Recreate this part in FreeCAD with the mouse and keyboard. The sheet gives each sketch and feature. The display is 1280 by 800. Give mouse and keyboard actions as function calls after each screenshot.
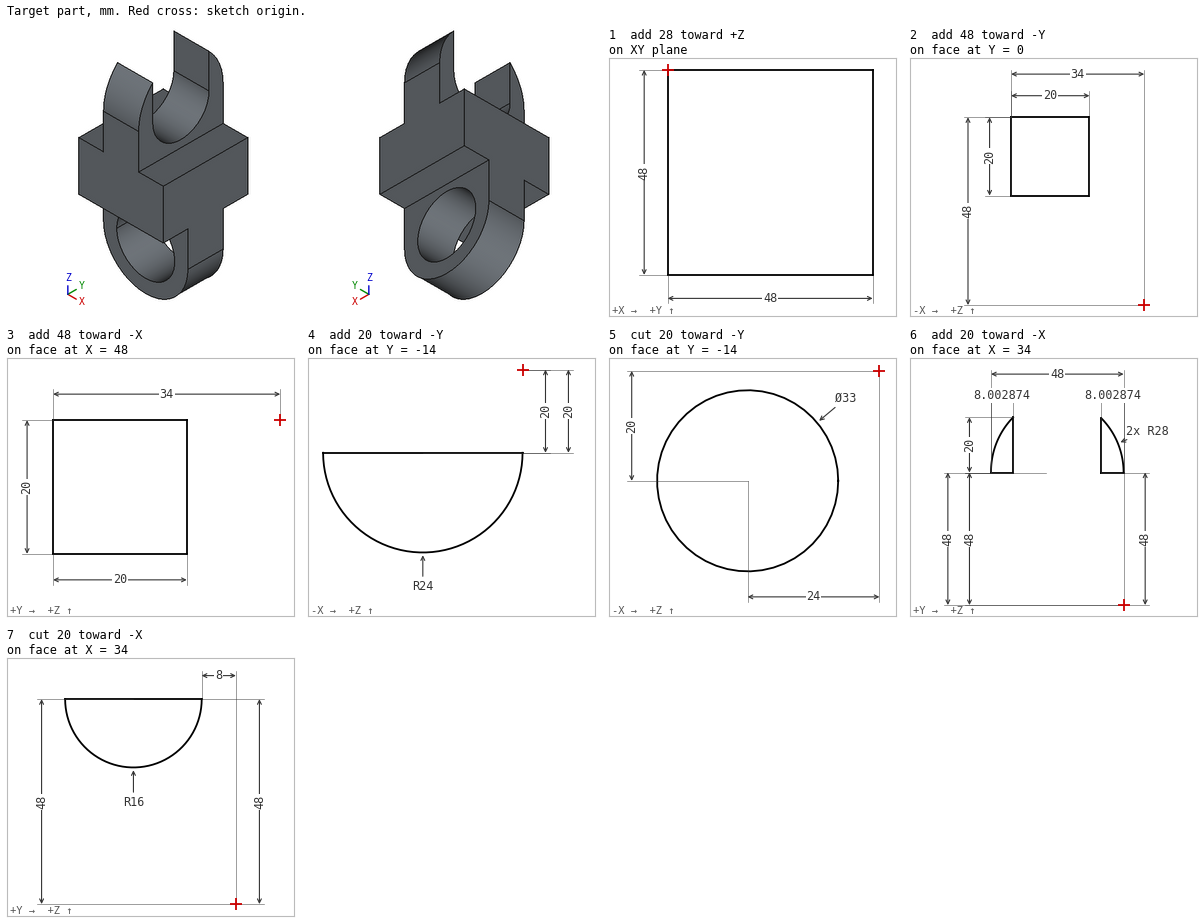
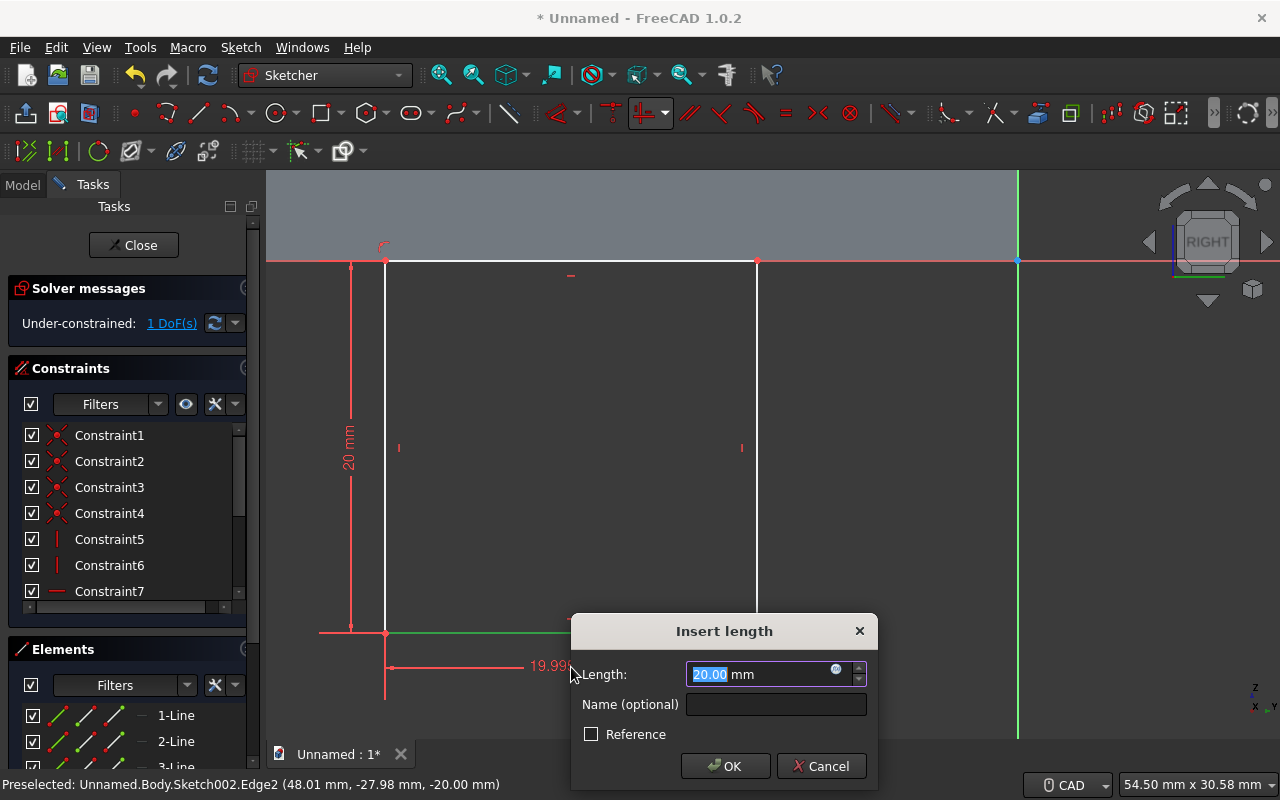
text(20)
key(Return)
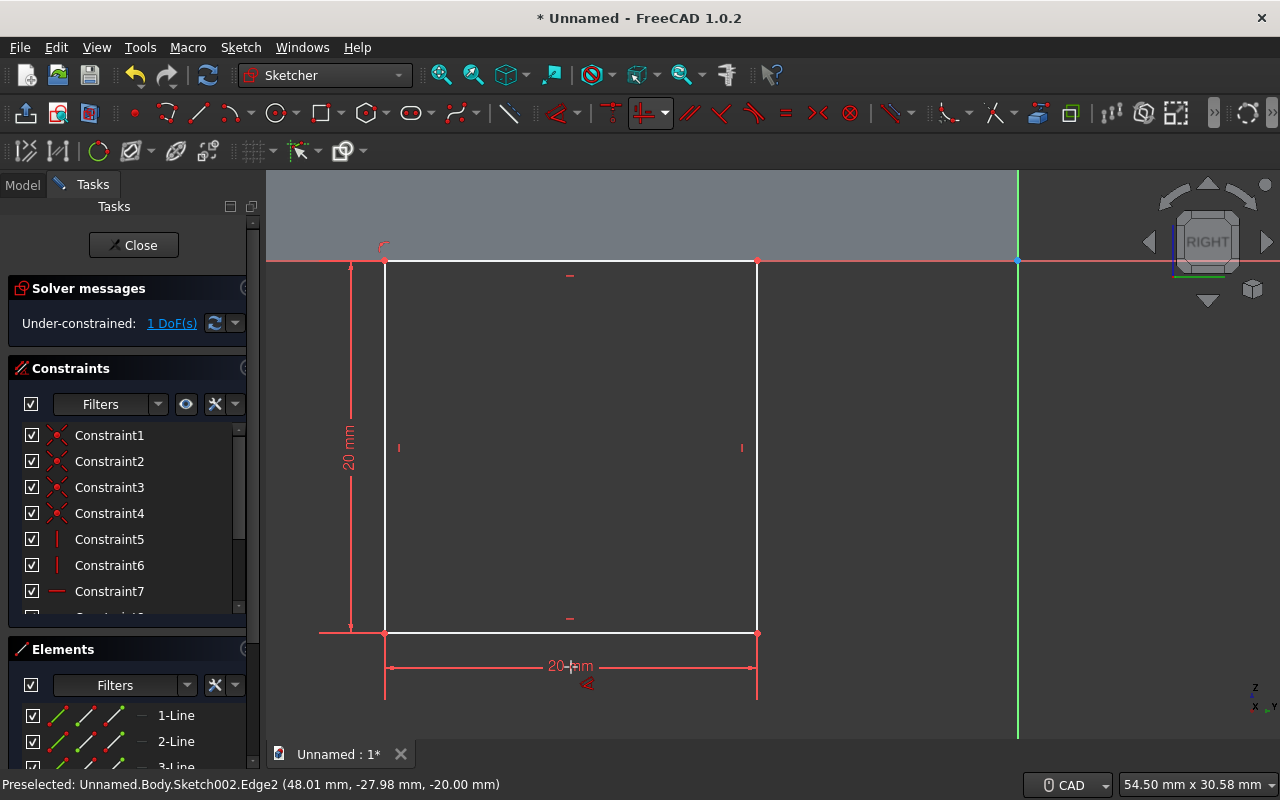
click(385, 261)
click(701, 227)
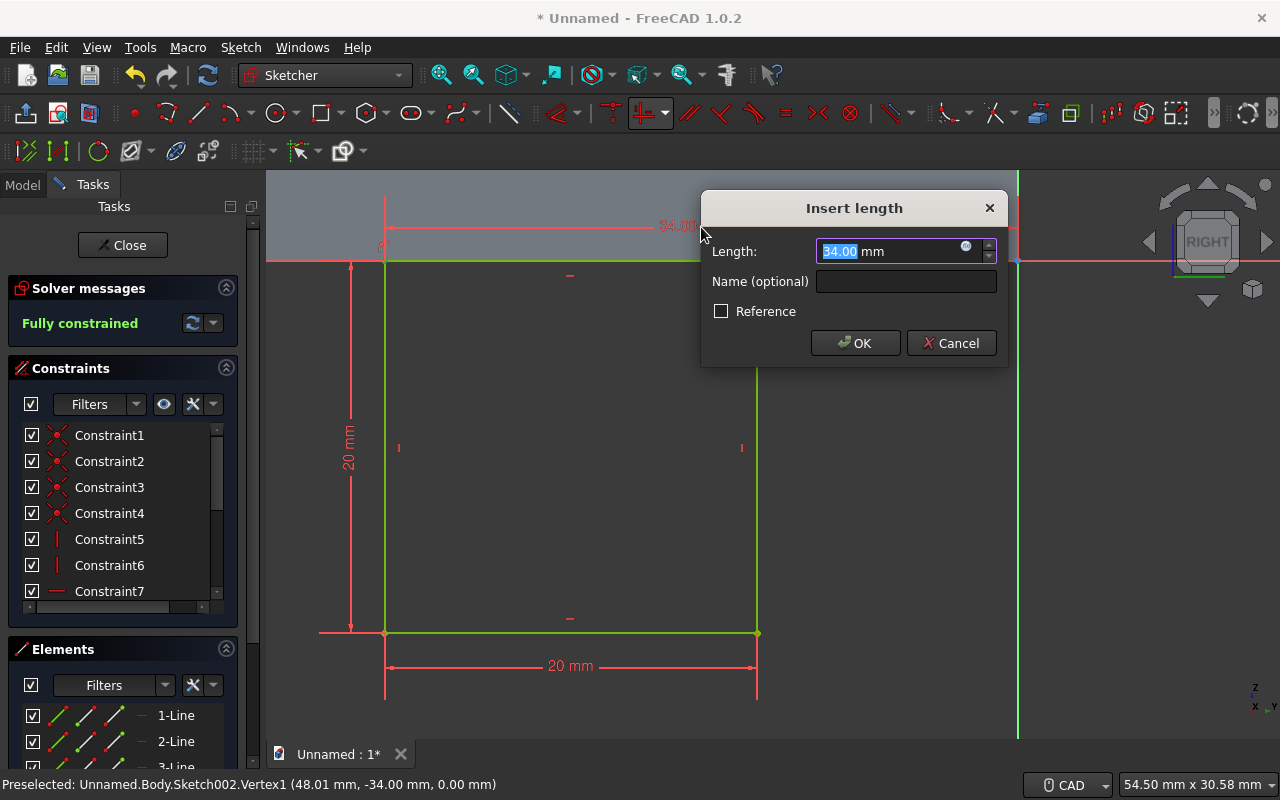
text(34)
key(Return)
key(Escape)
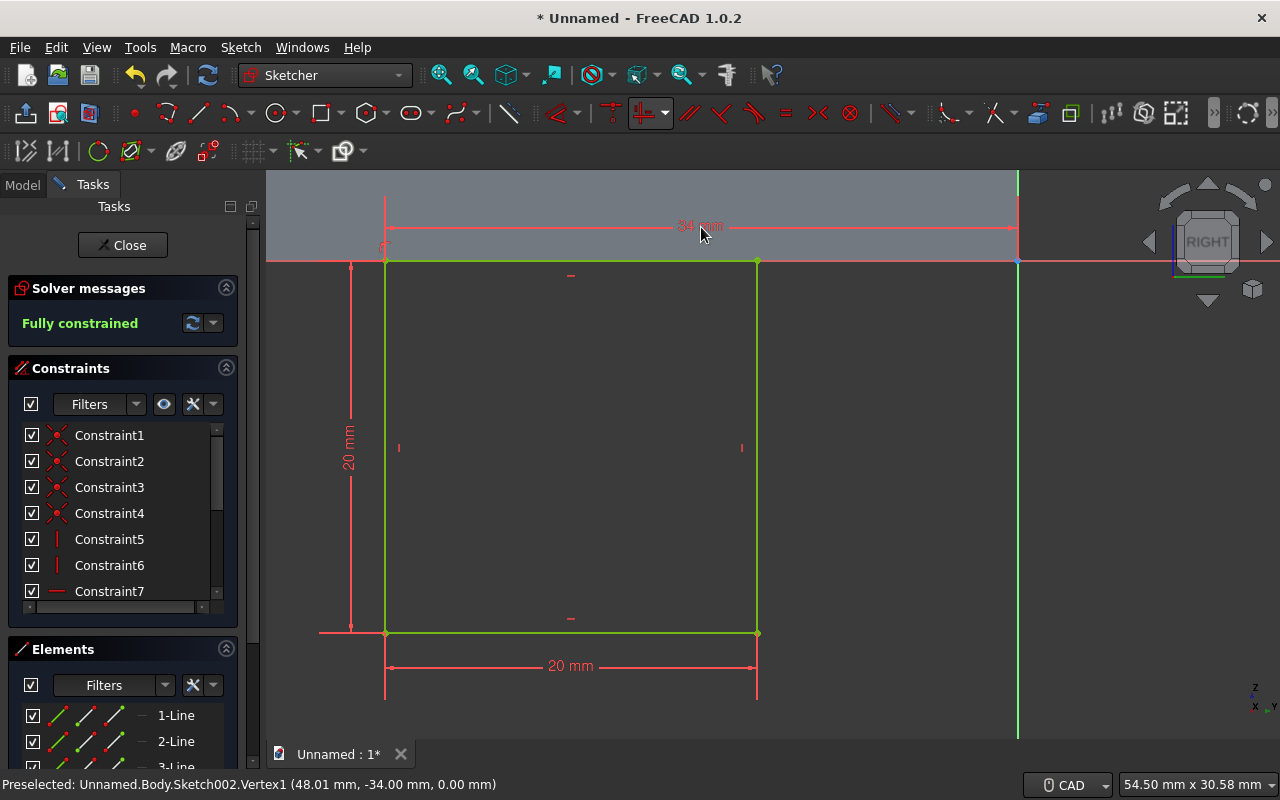
click(123, 245)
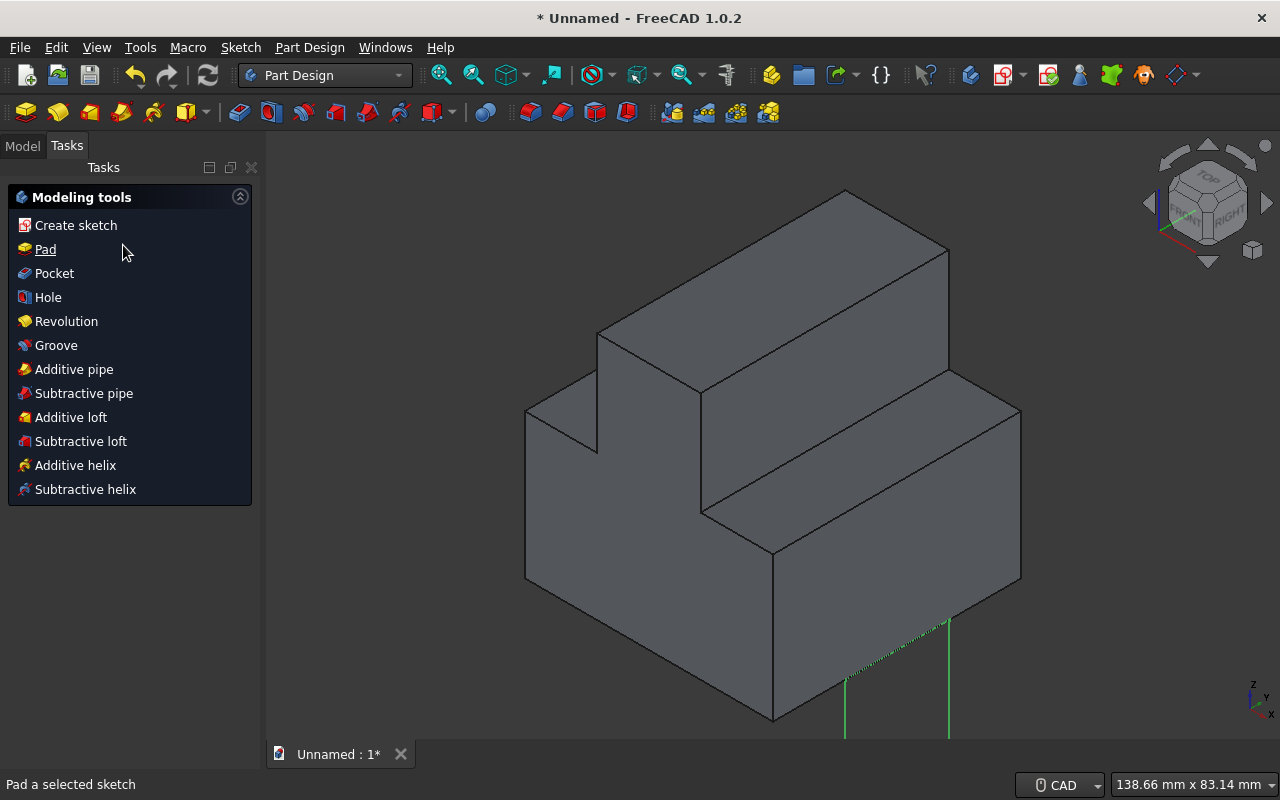
click(26, 112)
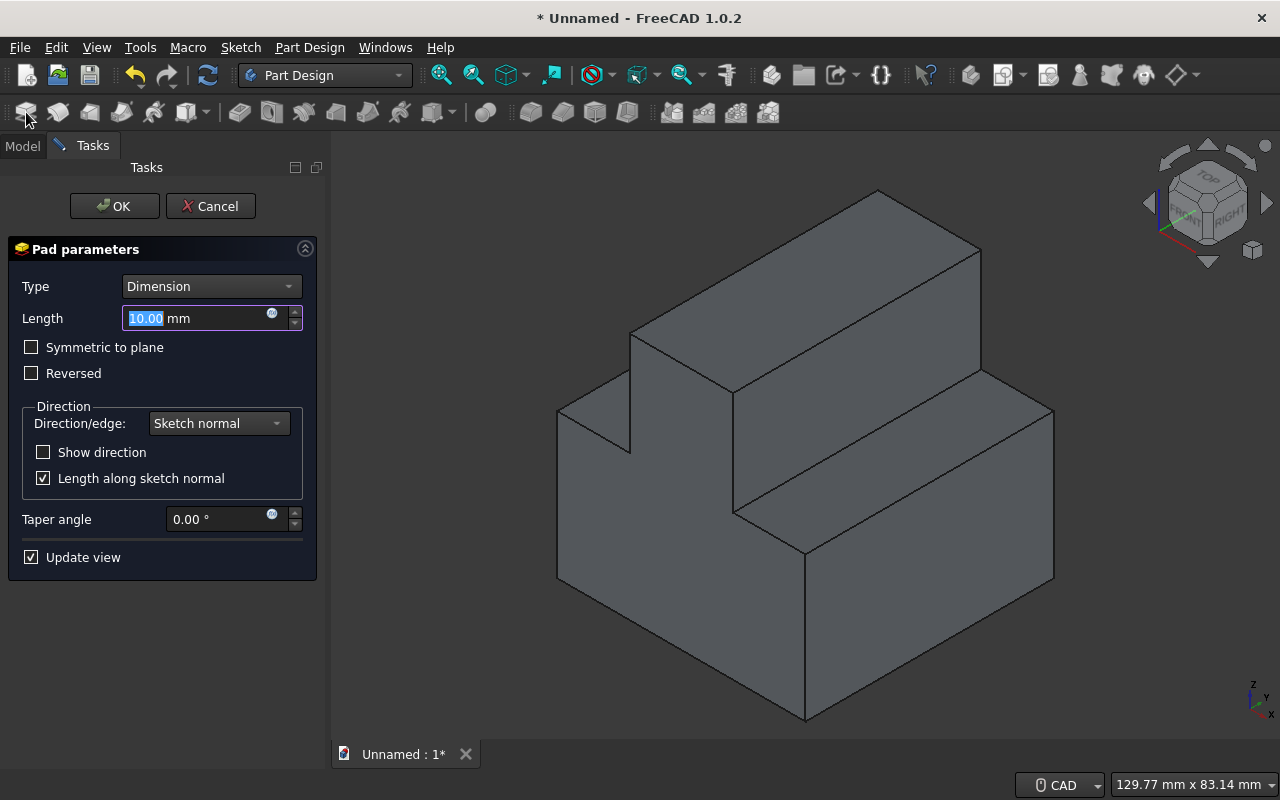
text(48)
key(Tab)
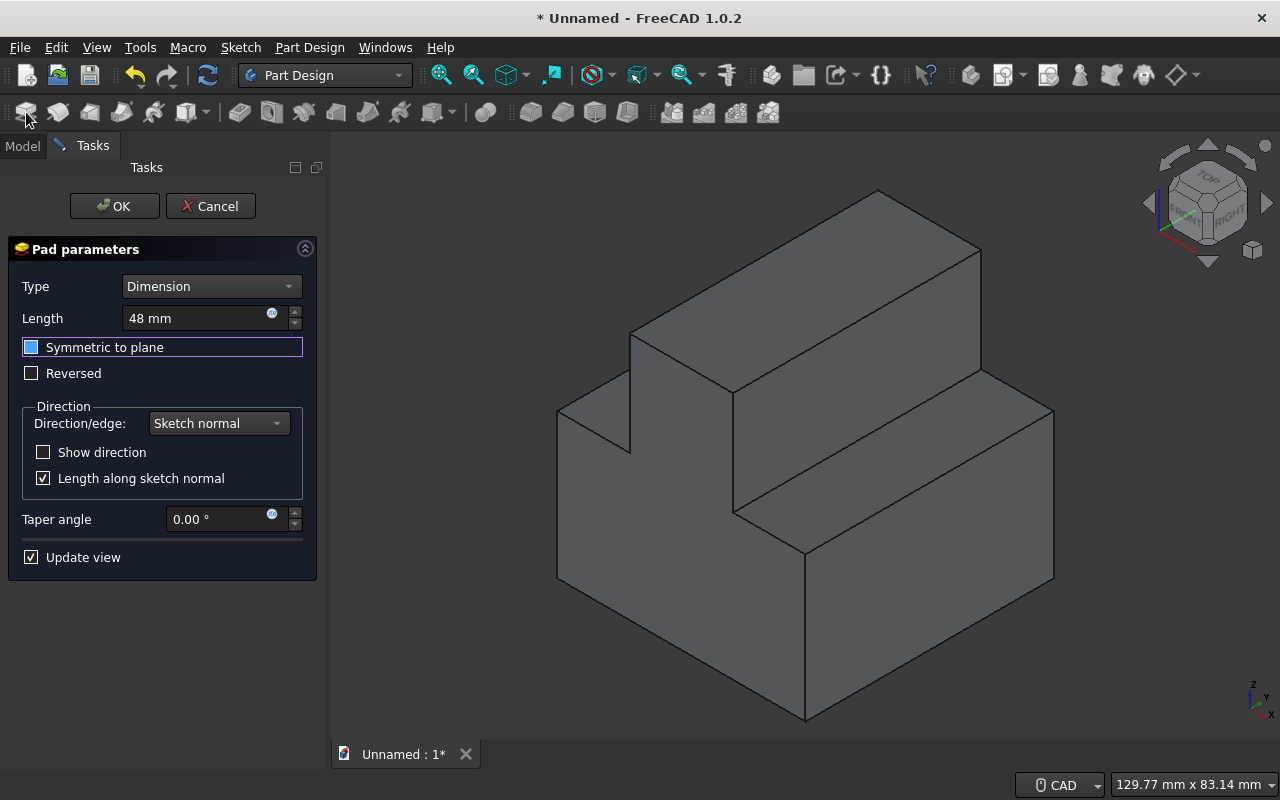
click(30, 373)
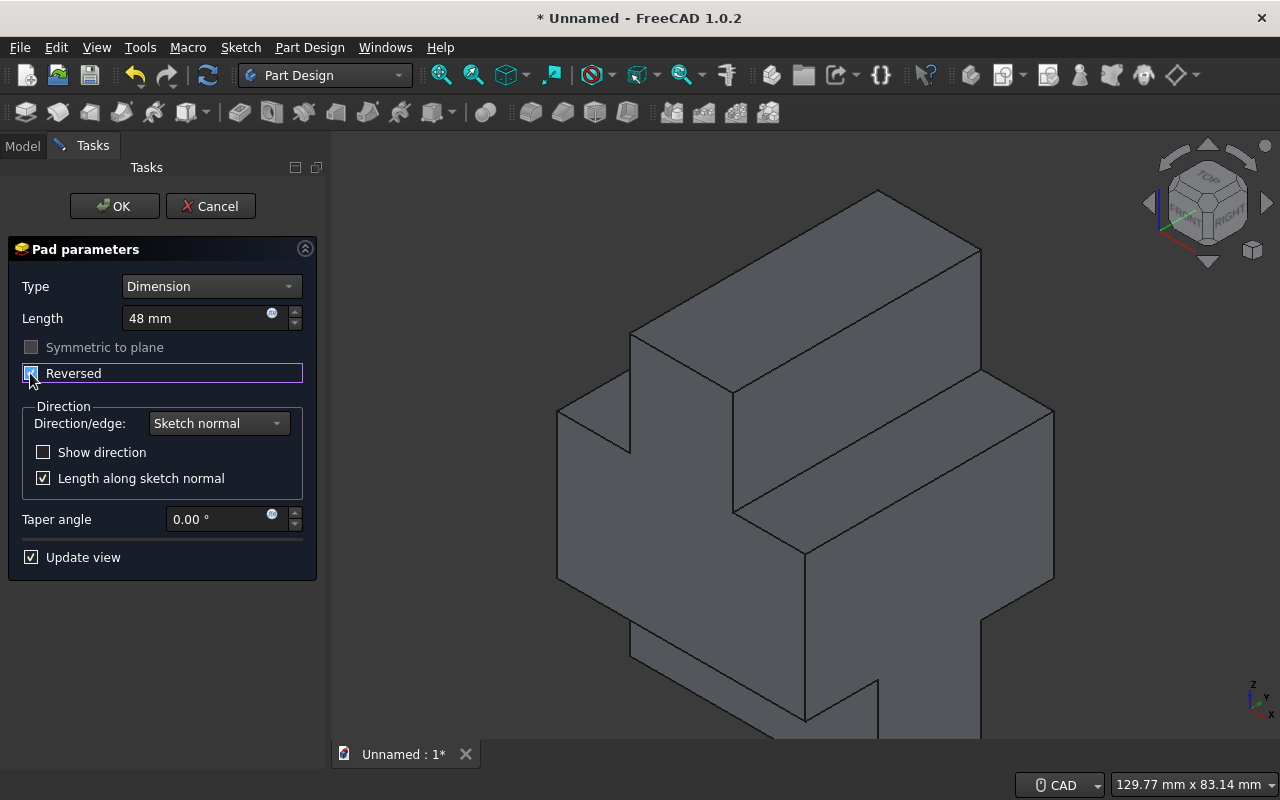
click(115, 206)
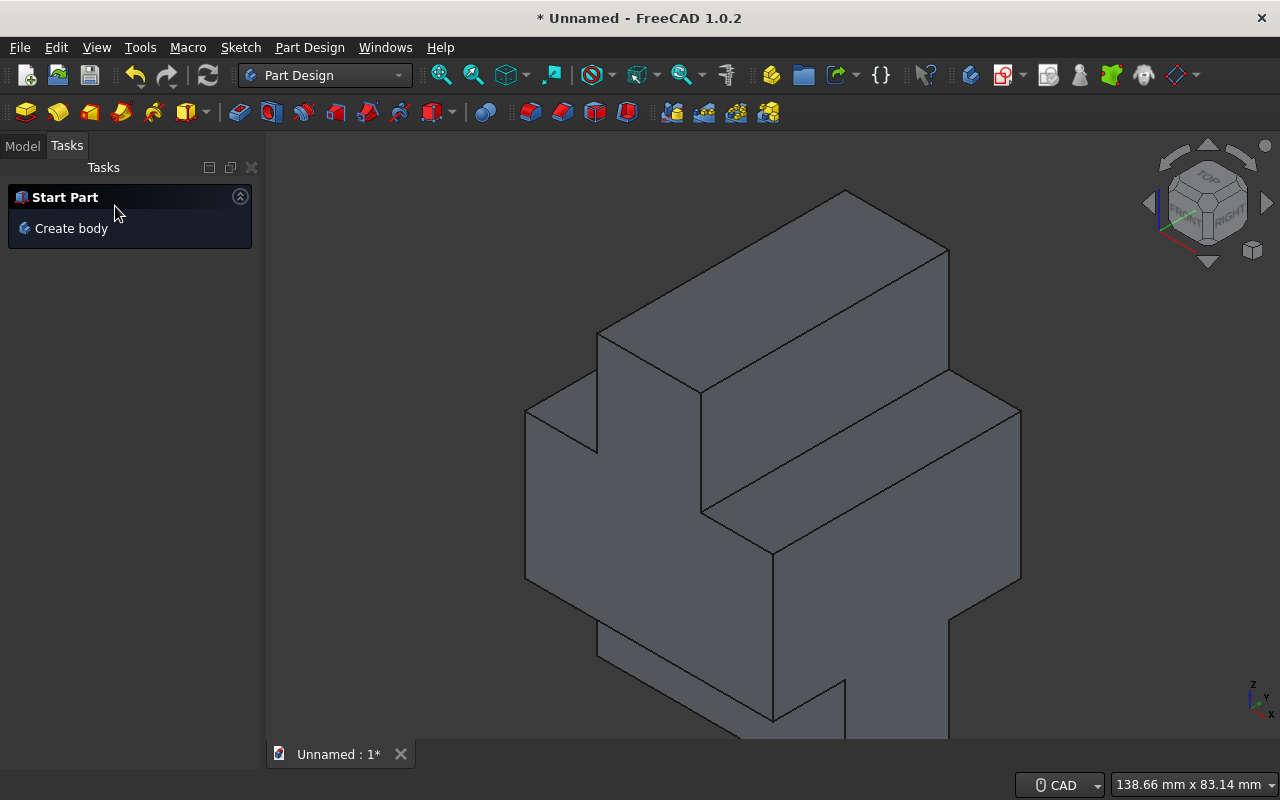
click(442, 76)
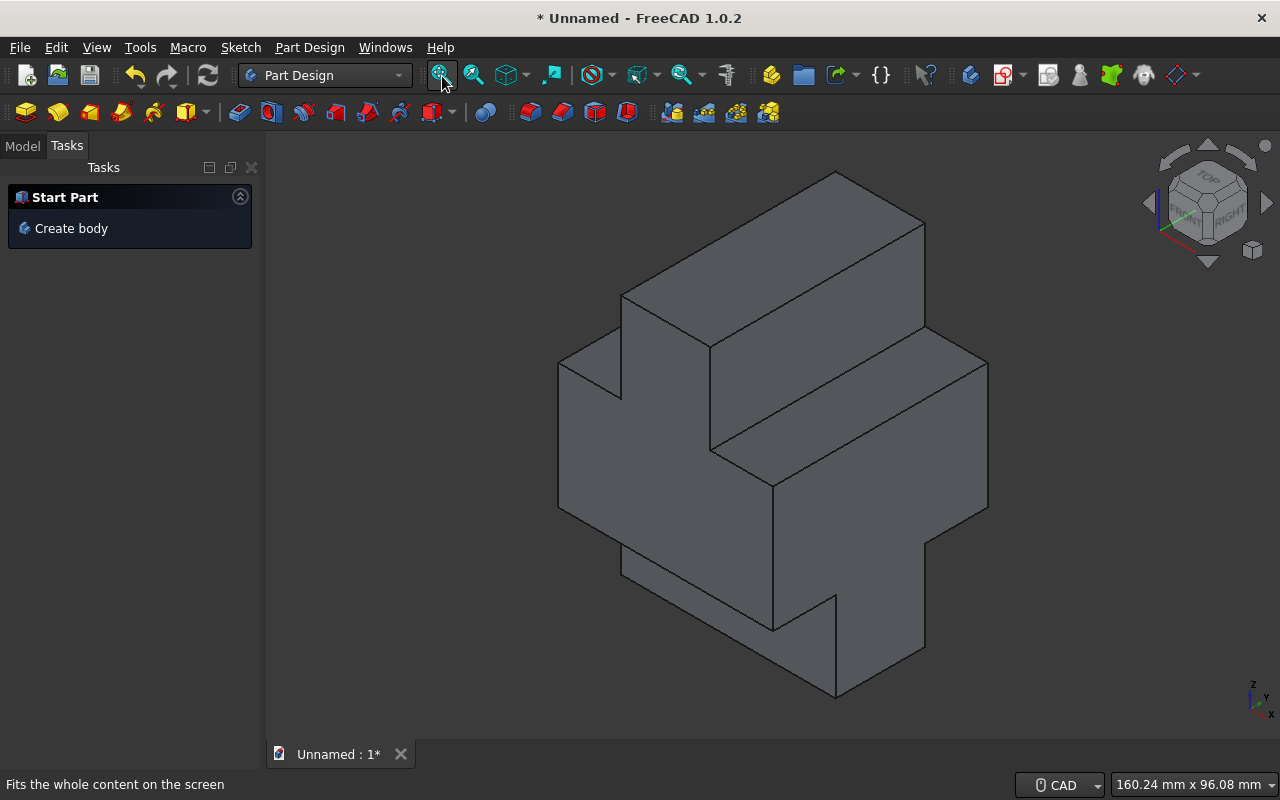
key(4)